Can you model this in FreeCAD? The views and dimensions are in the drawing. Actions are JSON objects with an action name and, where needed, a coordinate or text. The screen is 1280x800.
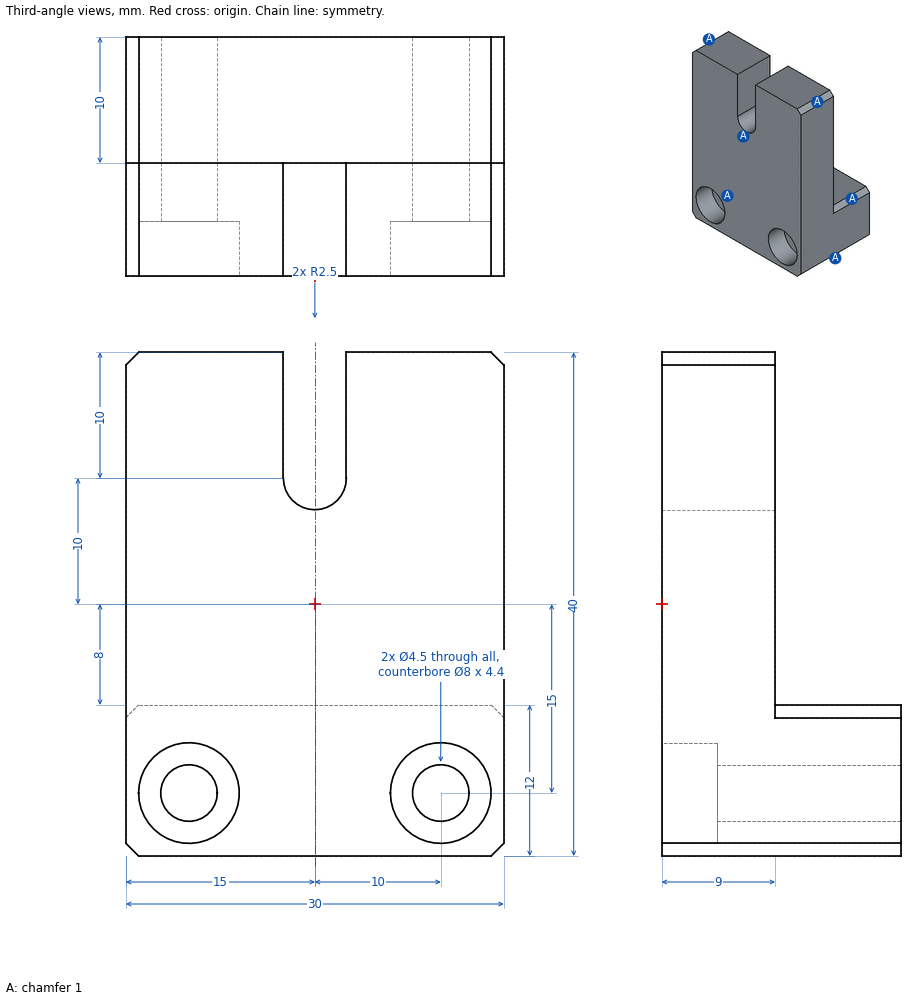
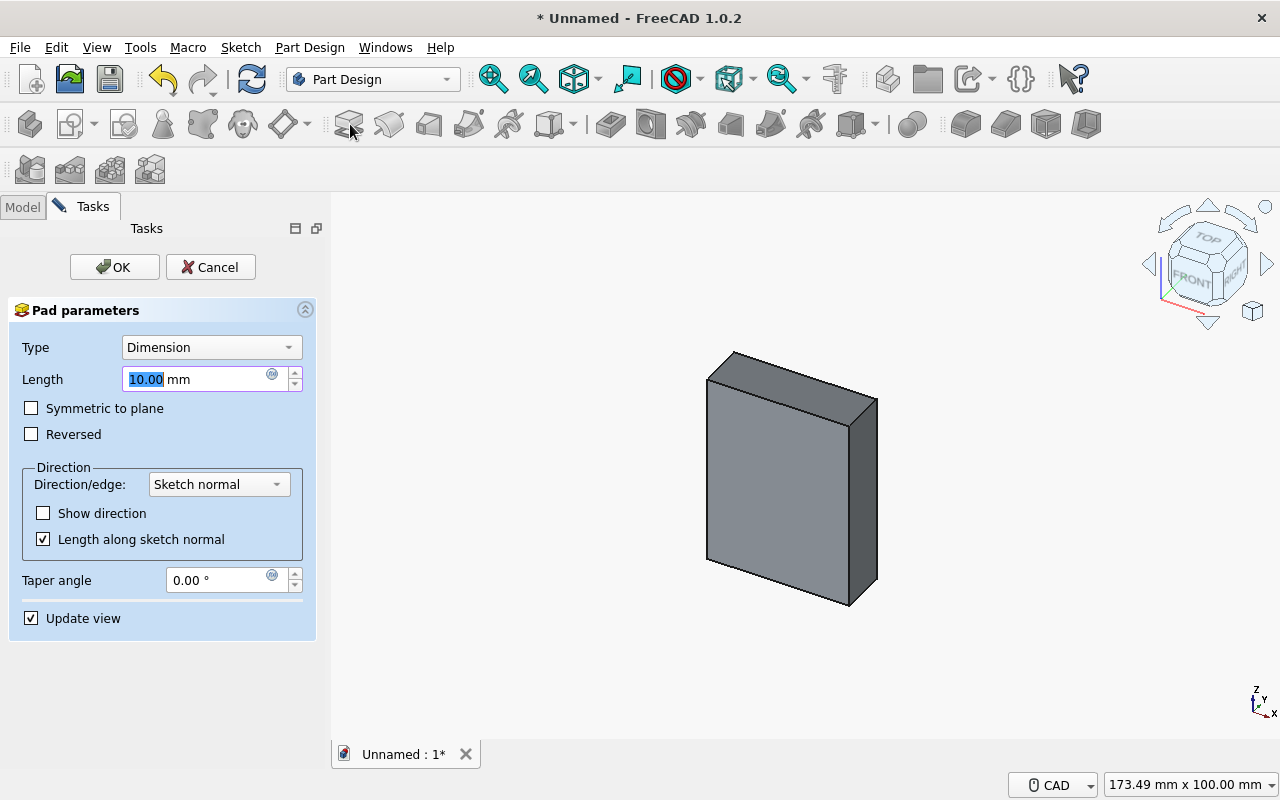
{"action": "type", "text": "9"}
{"action": "key", "text": "Tab"}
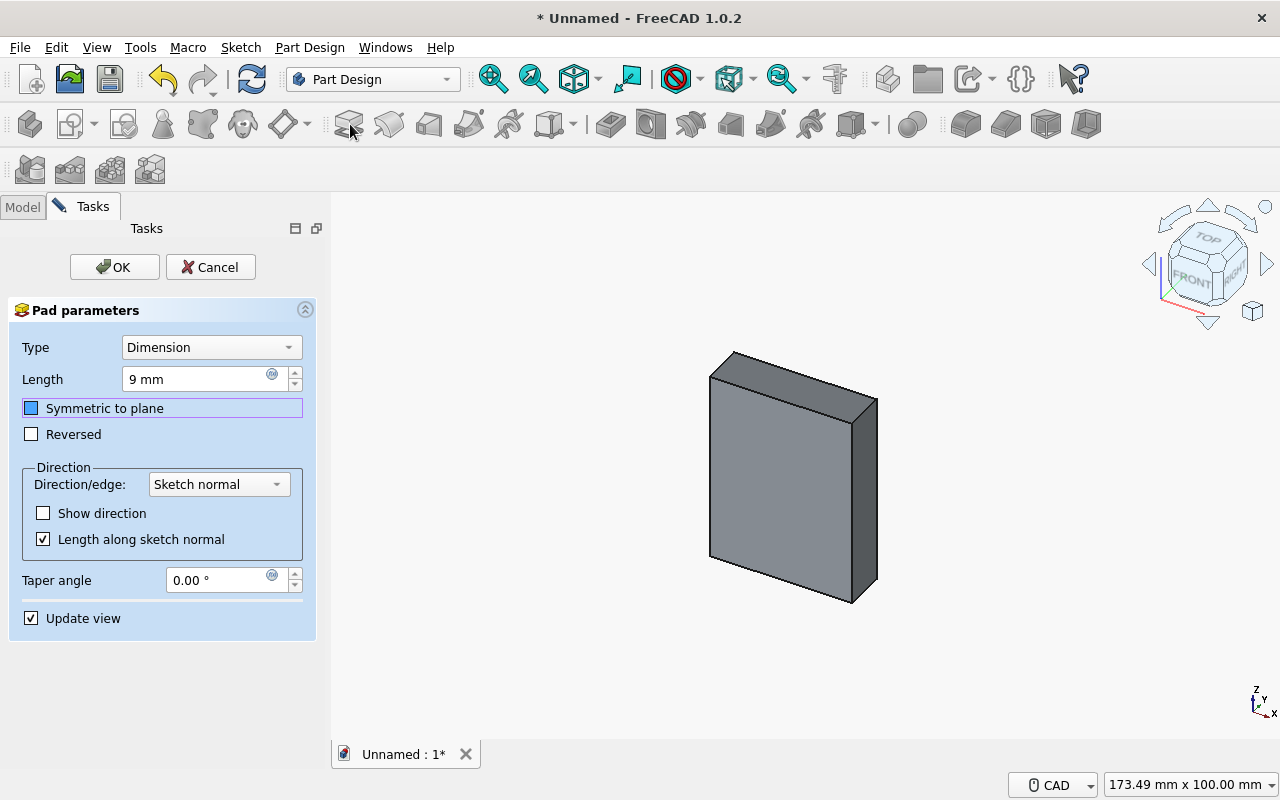
{"action": "left_click", "coordinate": [30, 434]}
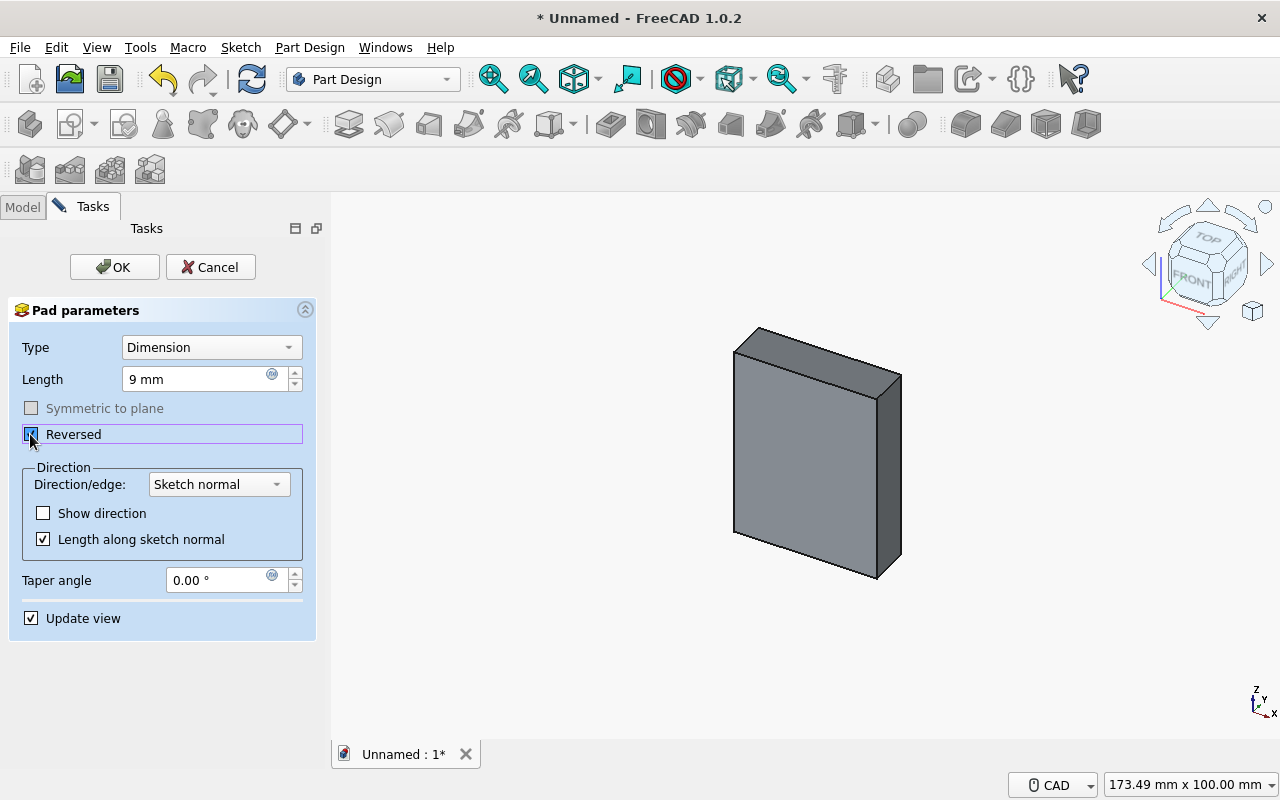
{"action": "left_click", "coordinate": [115, 267]}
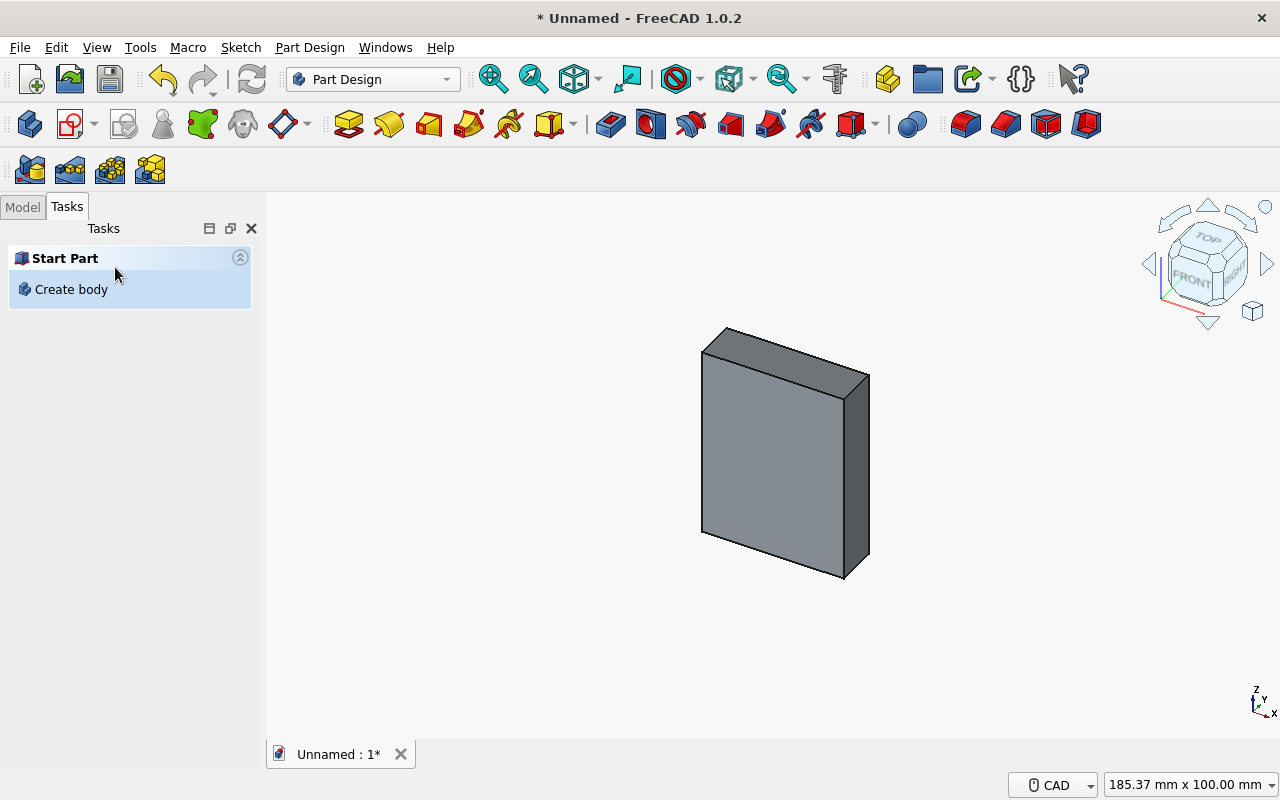
{"action": "key", "text": "4"}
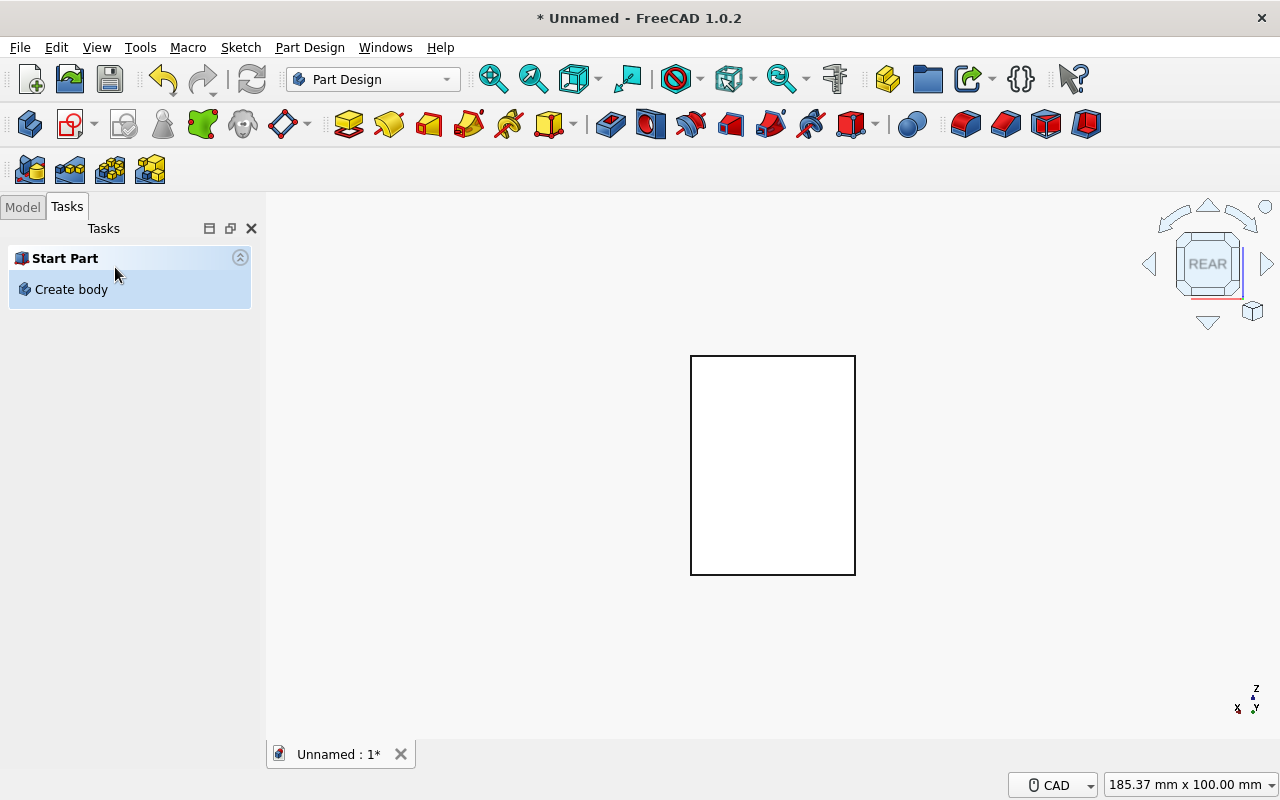
{"action": "key", "text": "v f"}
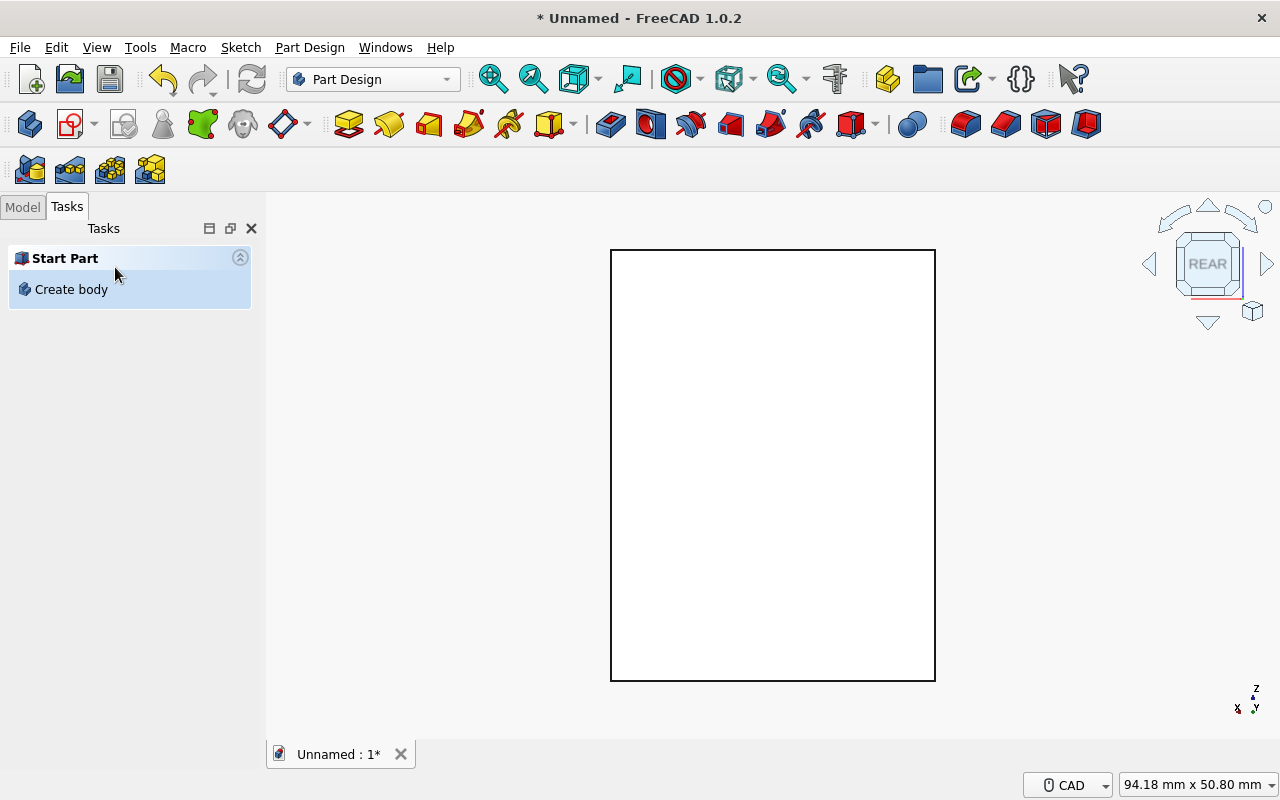
{"action": "left_click", "coordinate": [773, 465]}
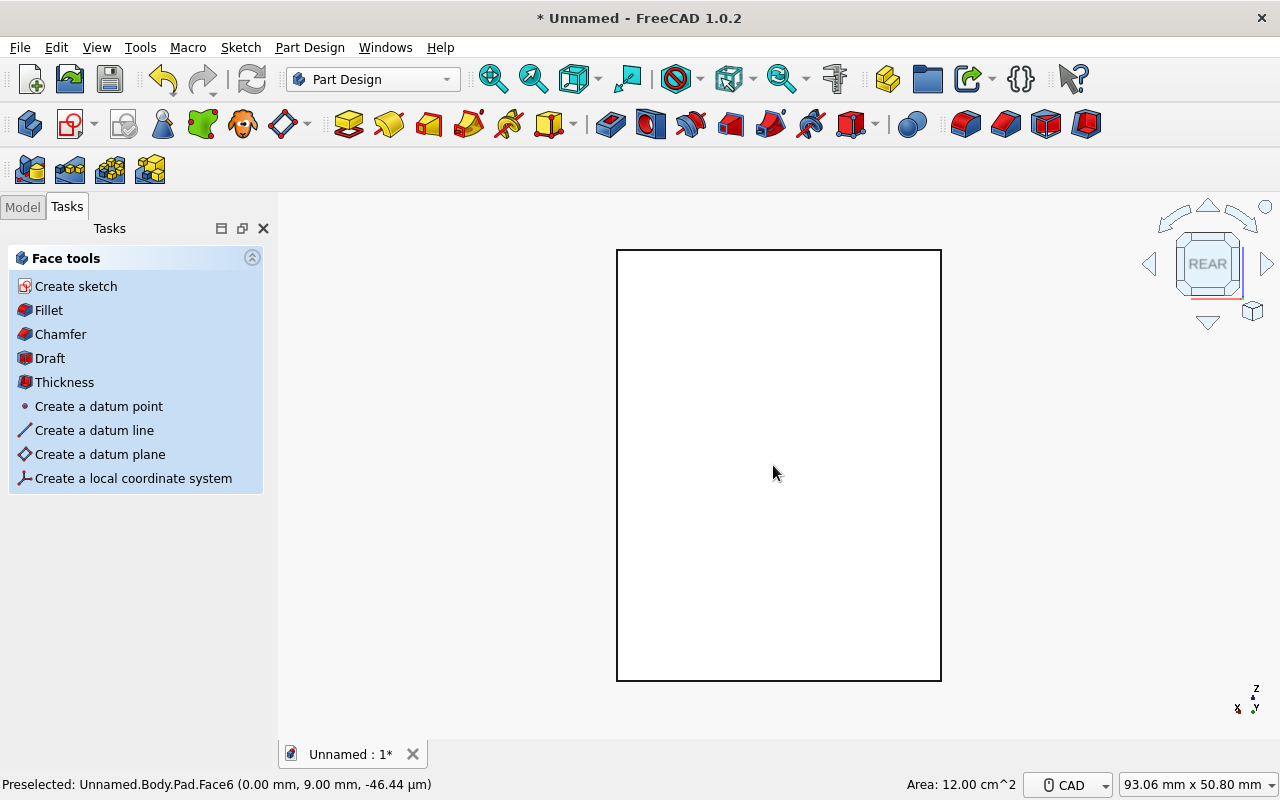
{"action": "left_click", "coordinate": [70, 124]}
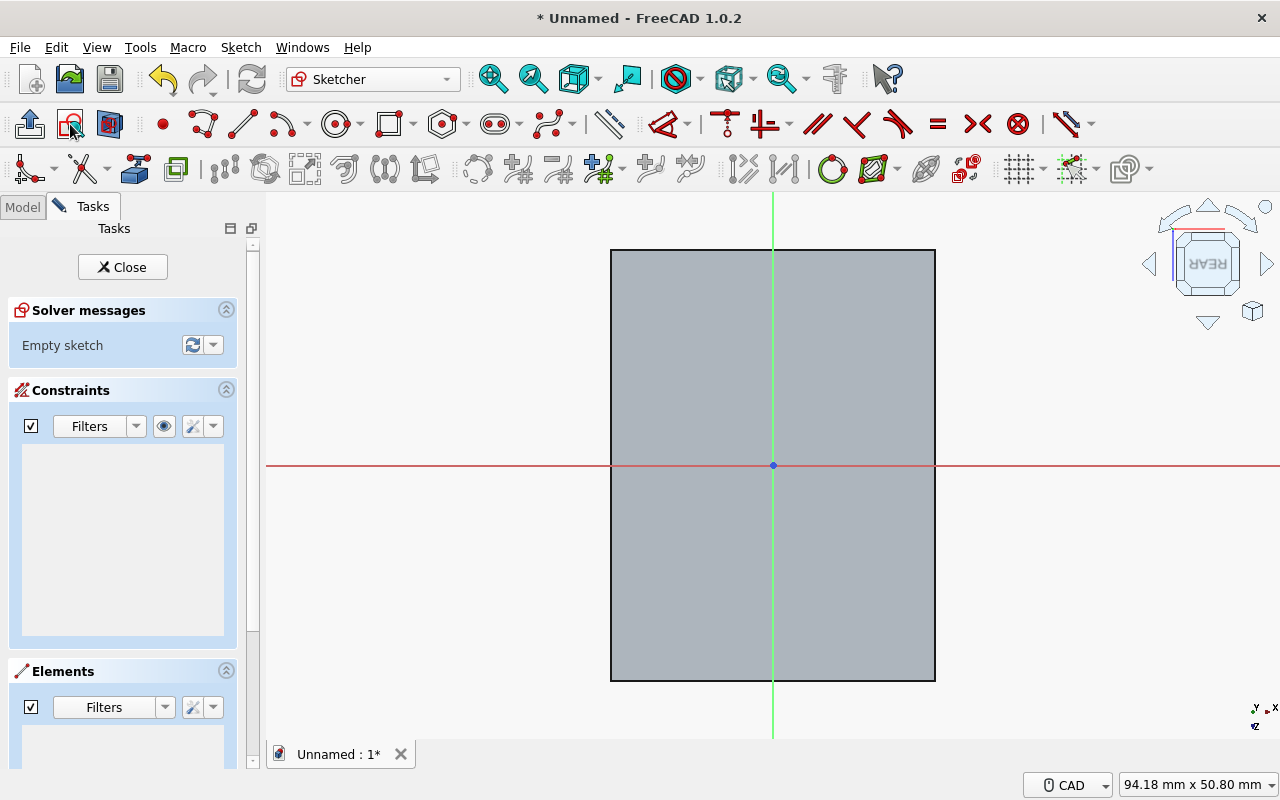
{"action": "scroll", "coordinate": [912, 220], "scroll_direction": "up", "scroll_amount": 2}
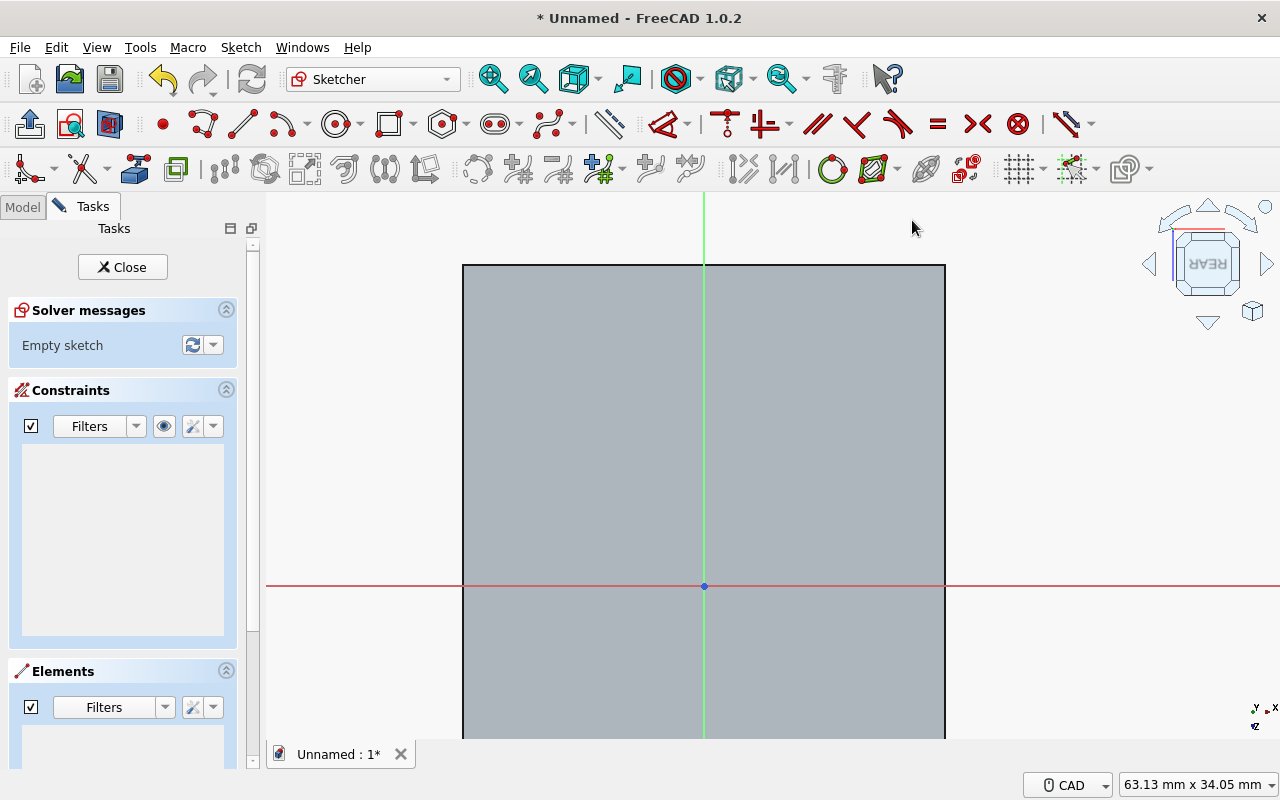
{"action": "left_click", "coordinate": [390, 124]}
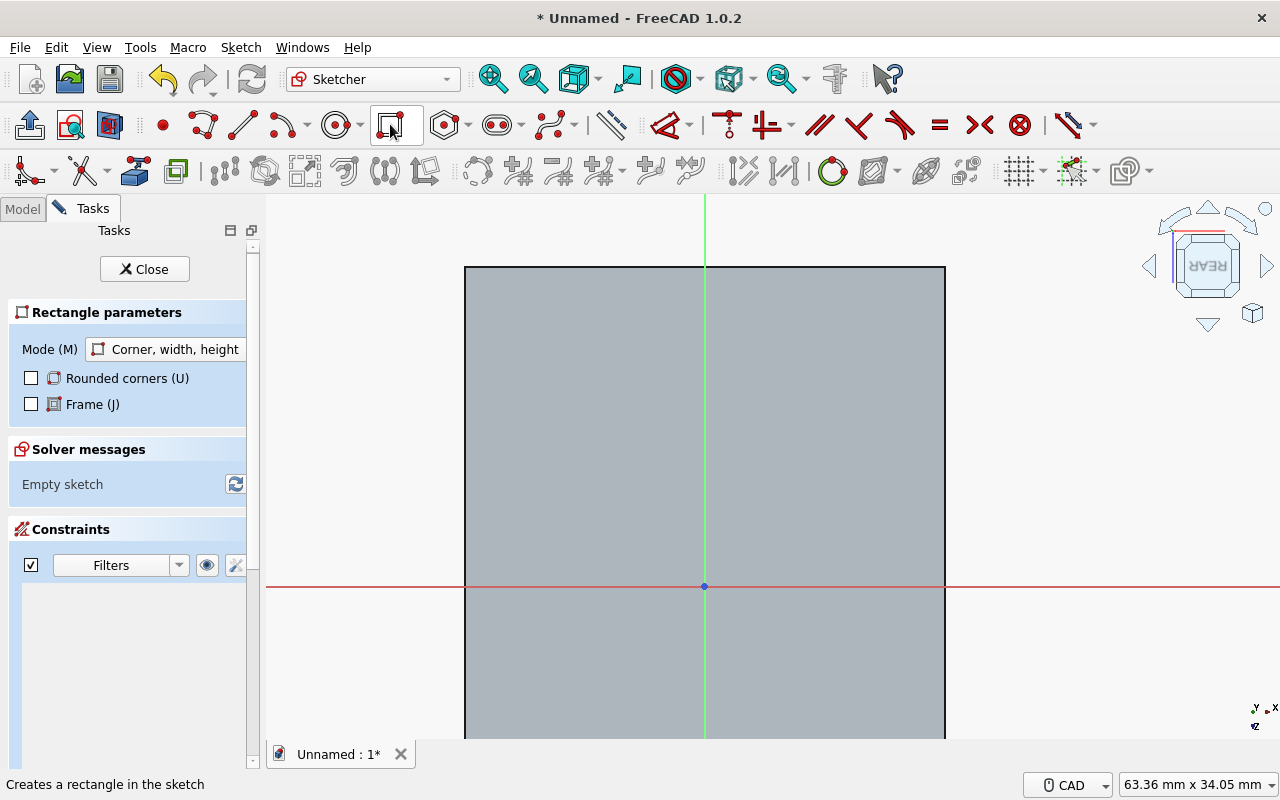
{"action": "left_click", "coordinate": [465, 267]}
{"action": "mouse_move", "coordinate": [945, 459]}